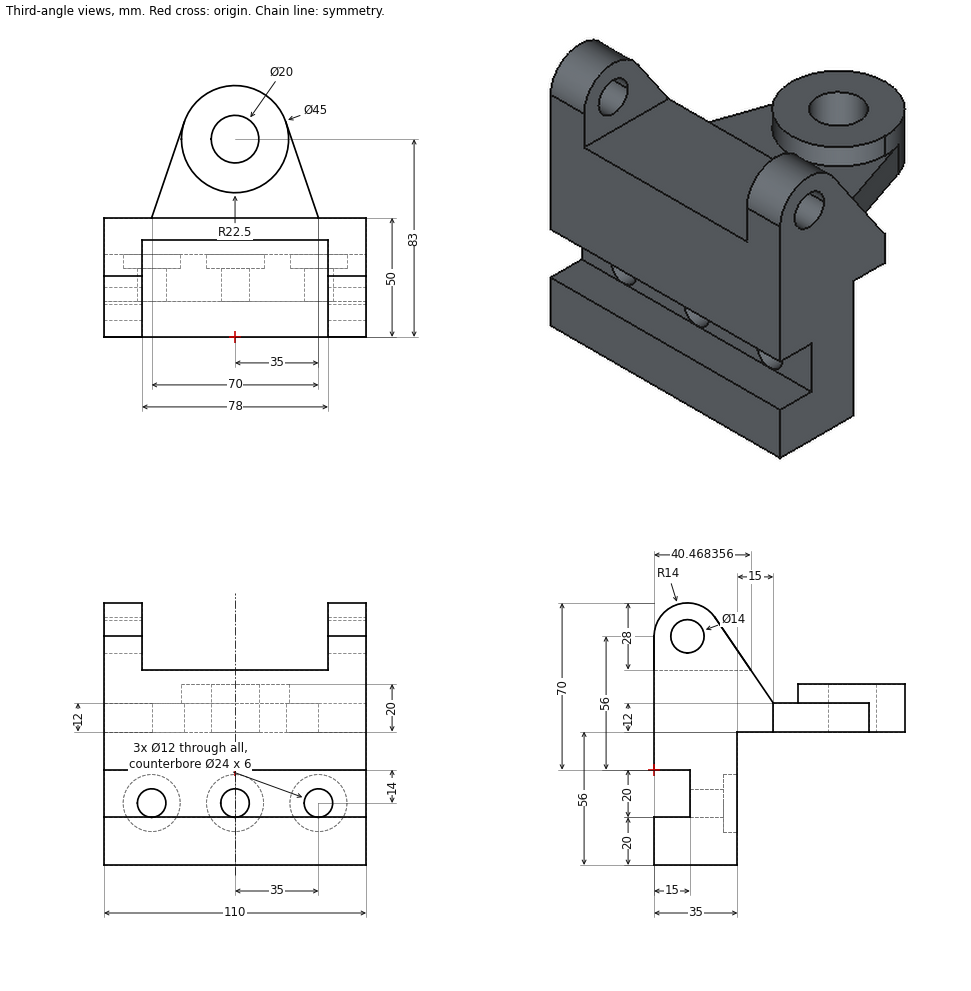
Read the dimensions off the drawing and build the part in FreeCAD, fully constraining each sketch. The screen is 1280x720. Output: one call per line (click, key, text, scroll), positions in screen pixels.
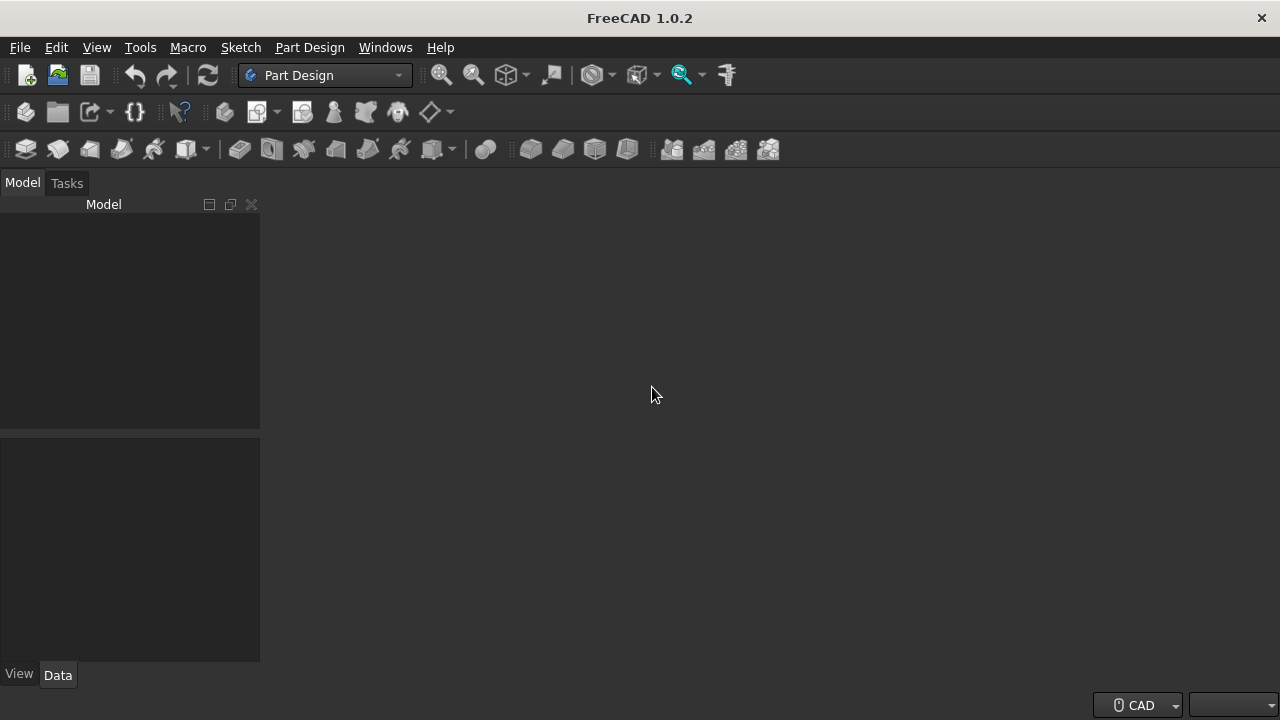
click(26, 76)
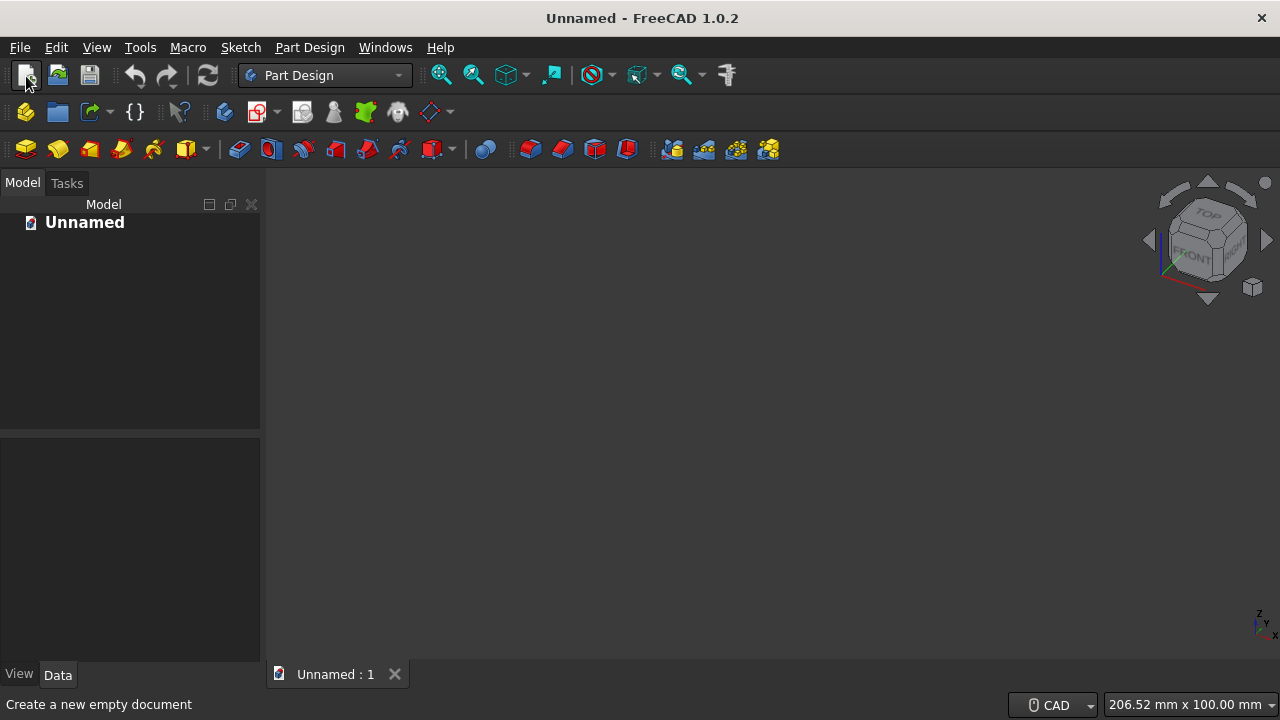
click(258, 112)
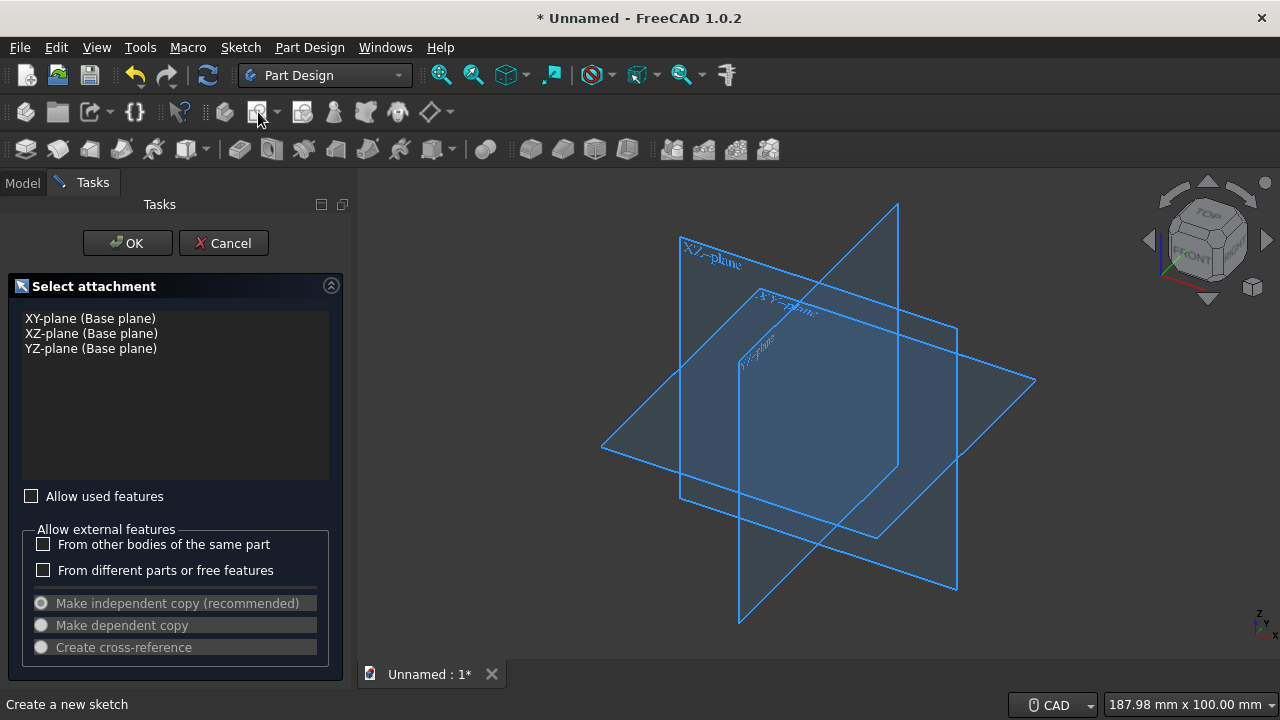
click(82, 348)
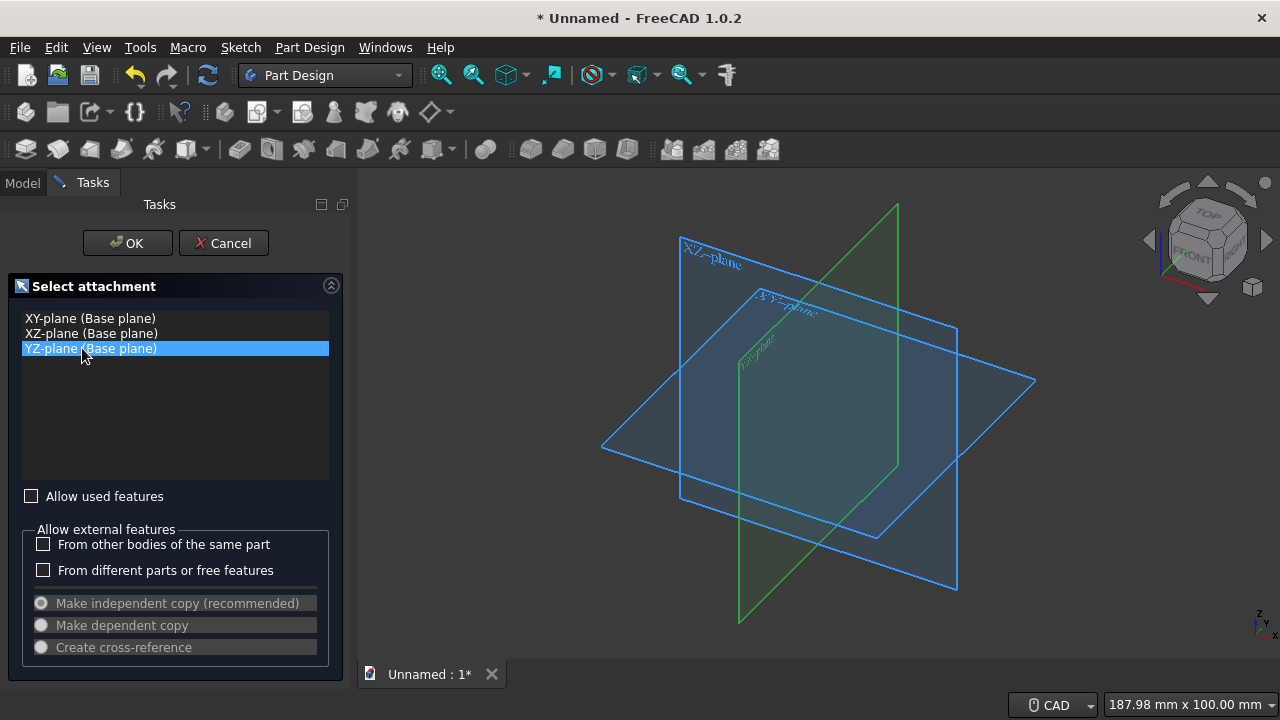
click(128, 243)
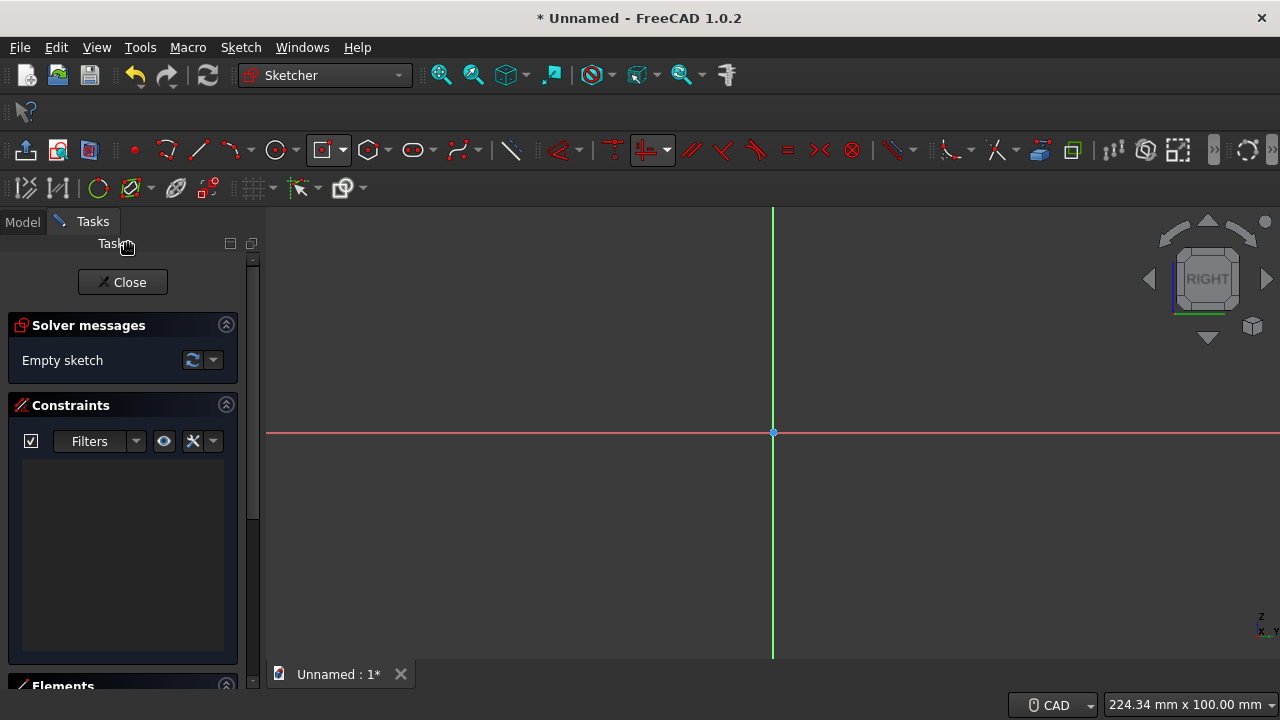
scroll(484, 514, down, 3)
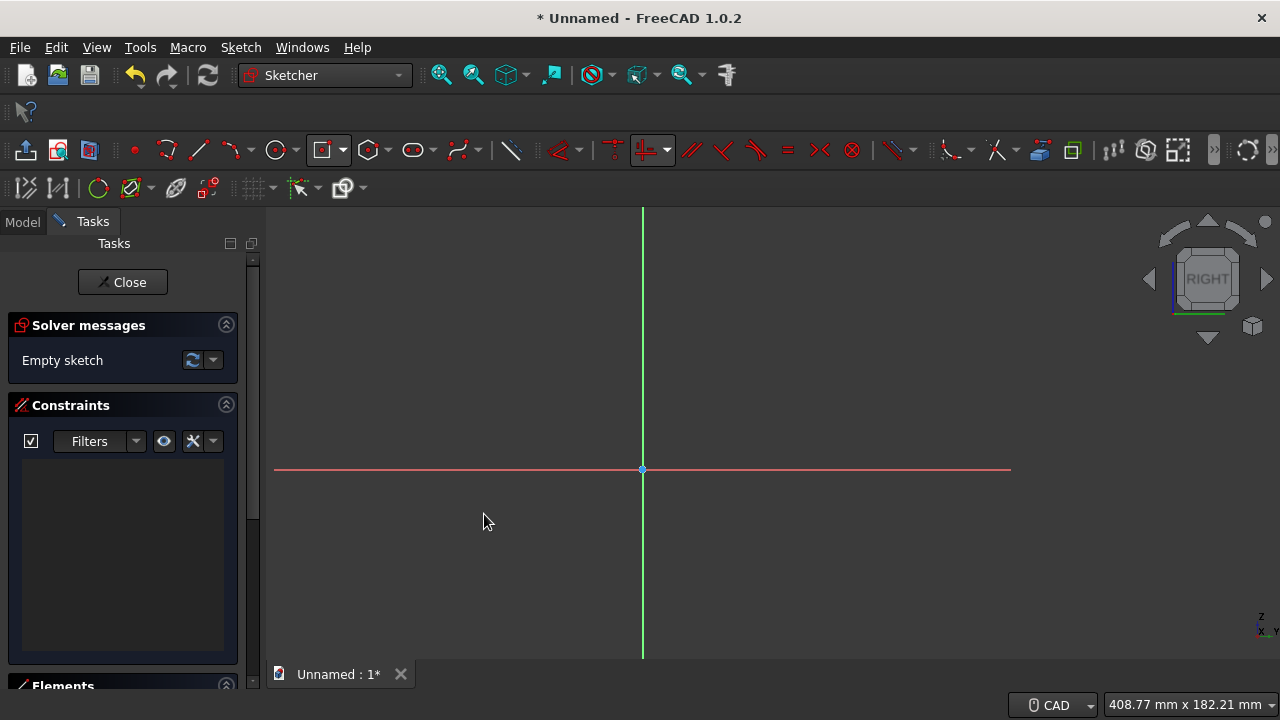
key(g)
key(m)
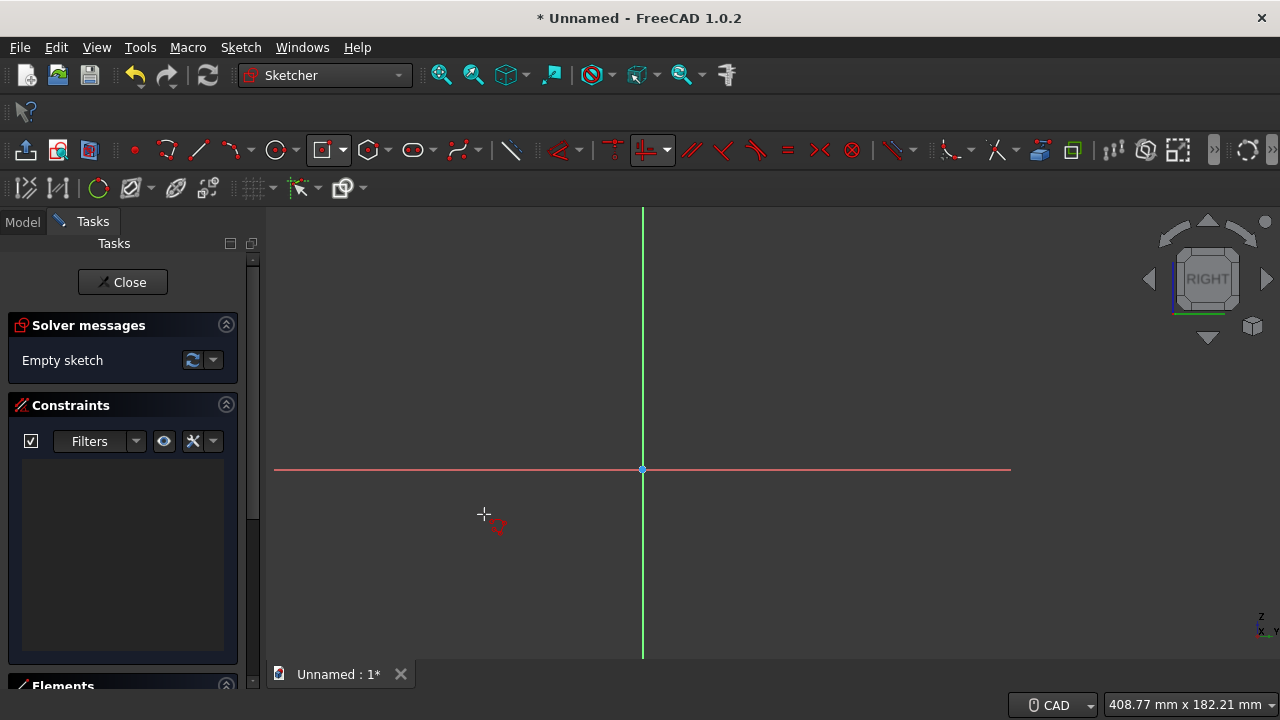
click(643, 331)
click(643, 470)
click(680, 461)
click(680, 519)
click(643, 519)
click(652, 569)
click(730, 569)
click(730, 430)
click(767, 430)
click(767, 400)
click(706, 311)
right_click(706, 311)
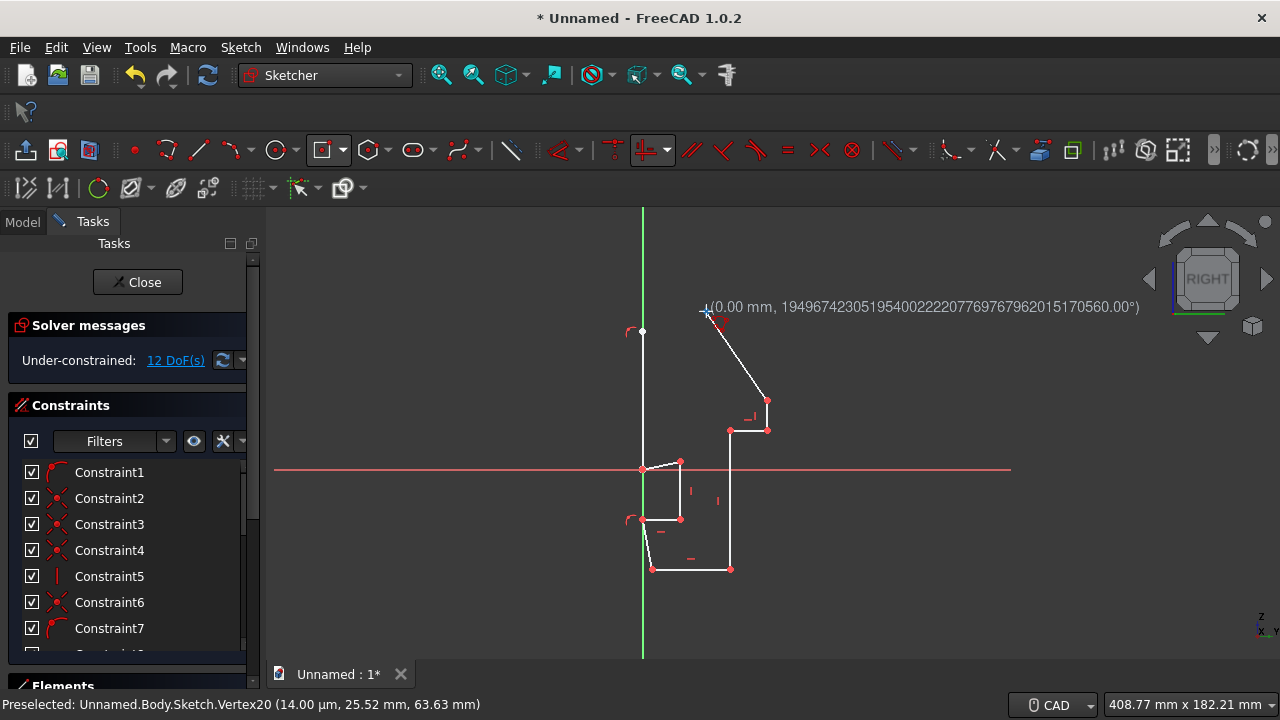
click(232, 150)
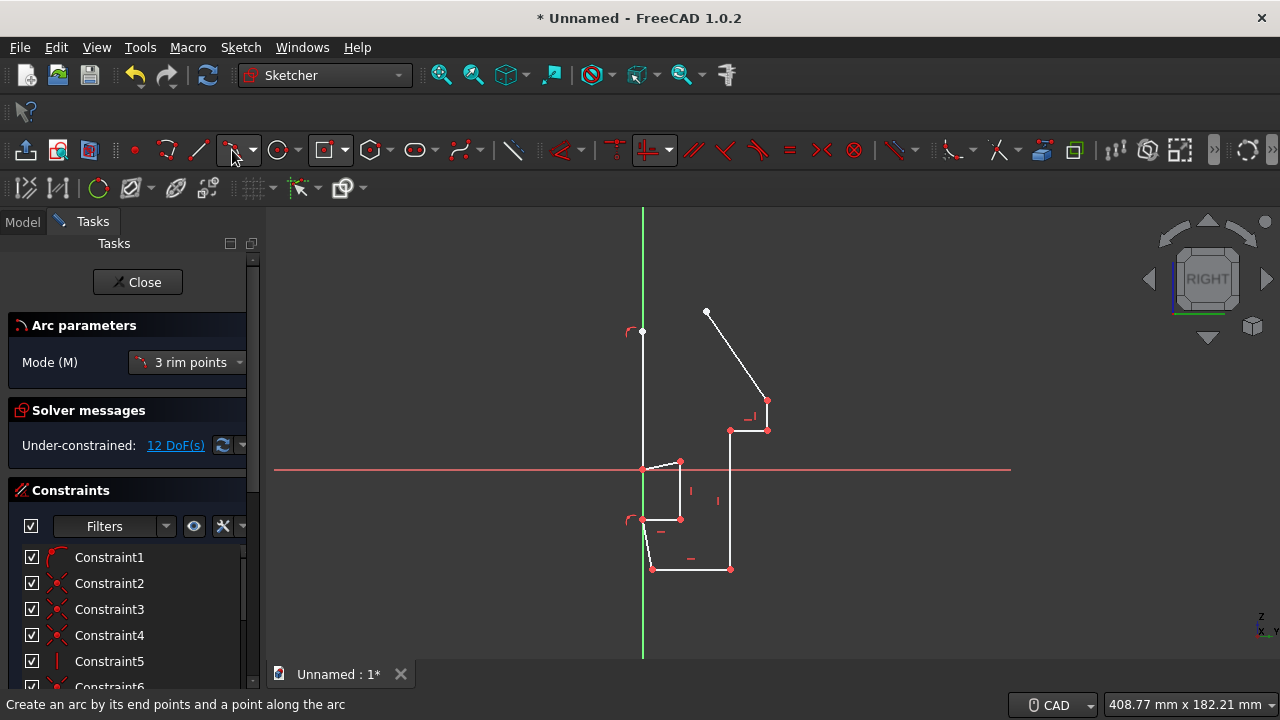
click(706, 312)
click(643, 332)
click(667, 298)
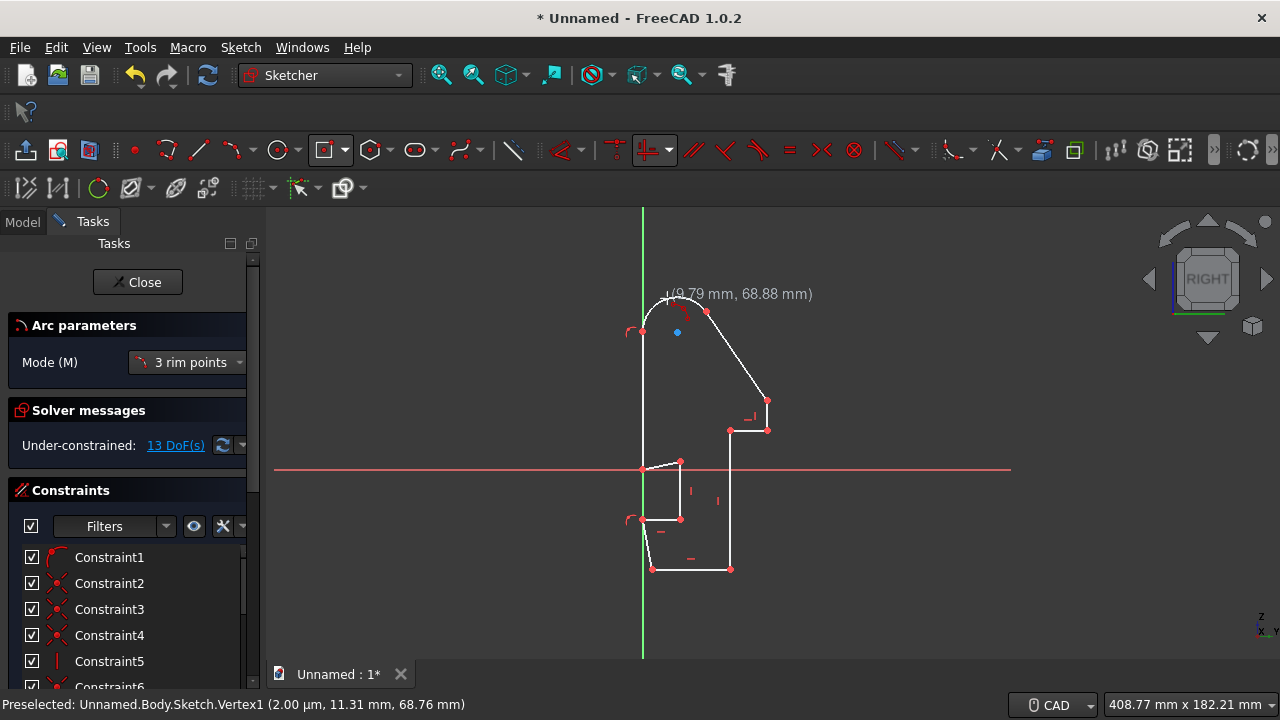
click(278, 150)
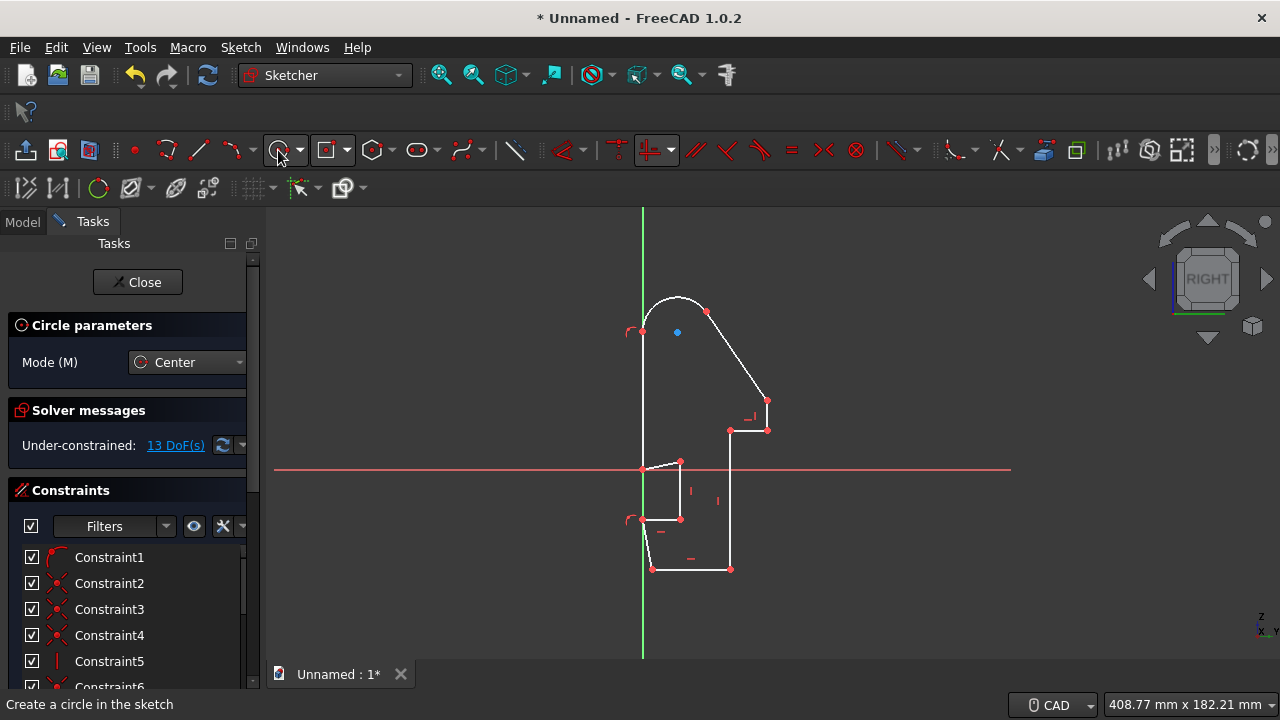
scroll(677, 331, up, 2)